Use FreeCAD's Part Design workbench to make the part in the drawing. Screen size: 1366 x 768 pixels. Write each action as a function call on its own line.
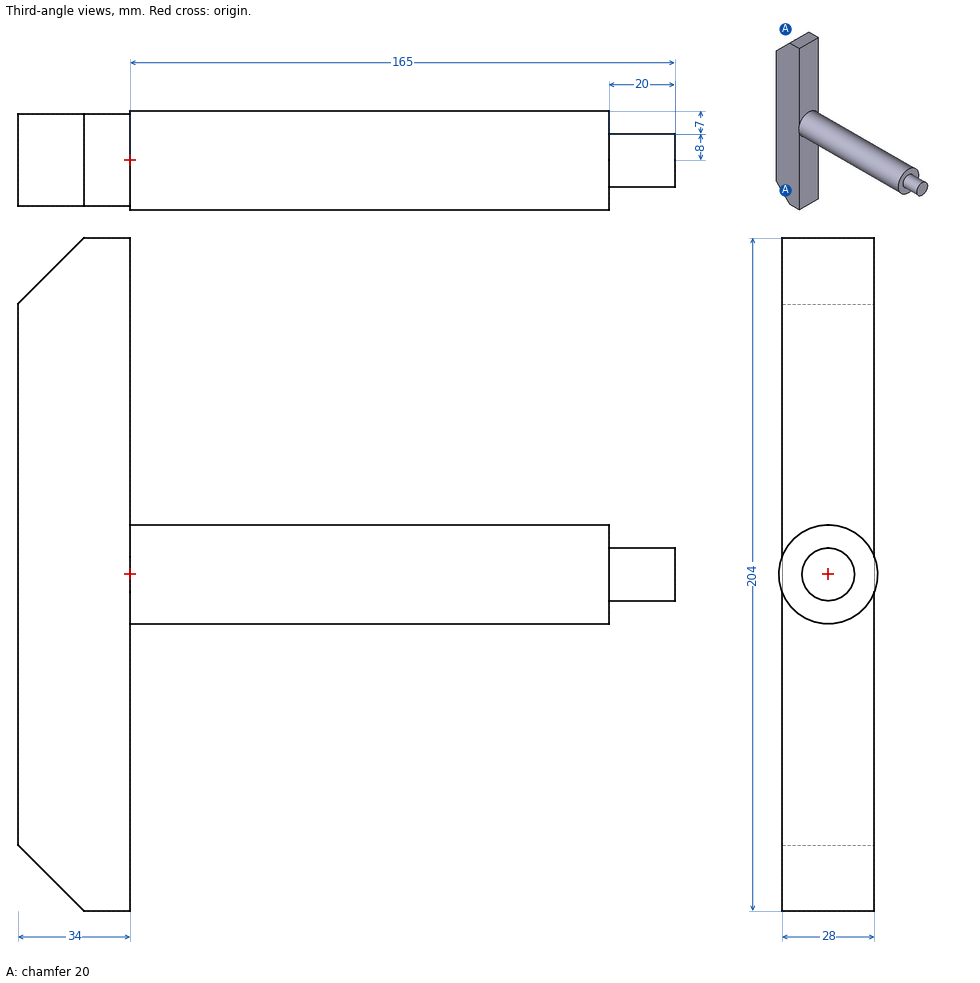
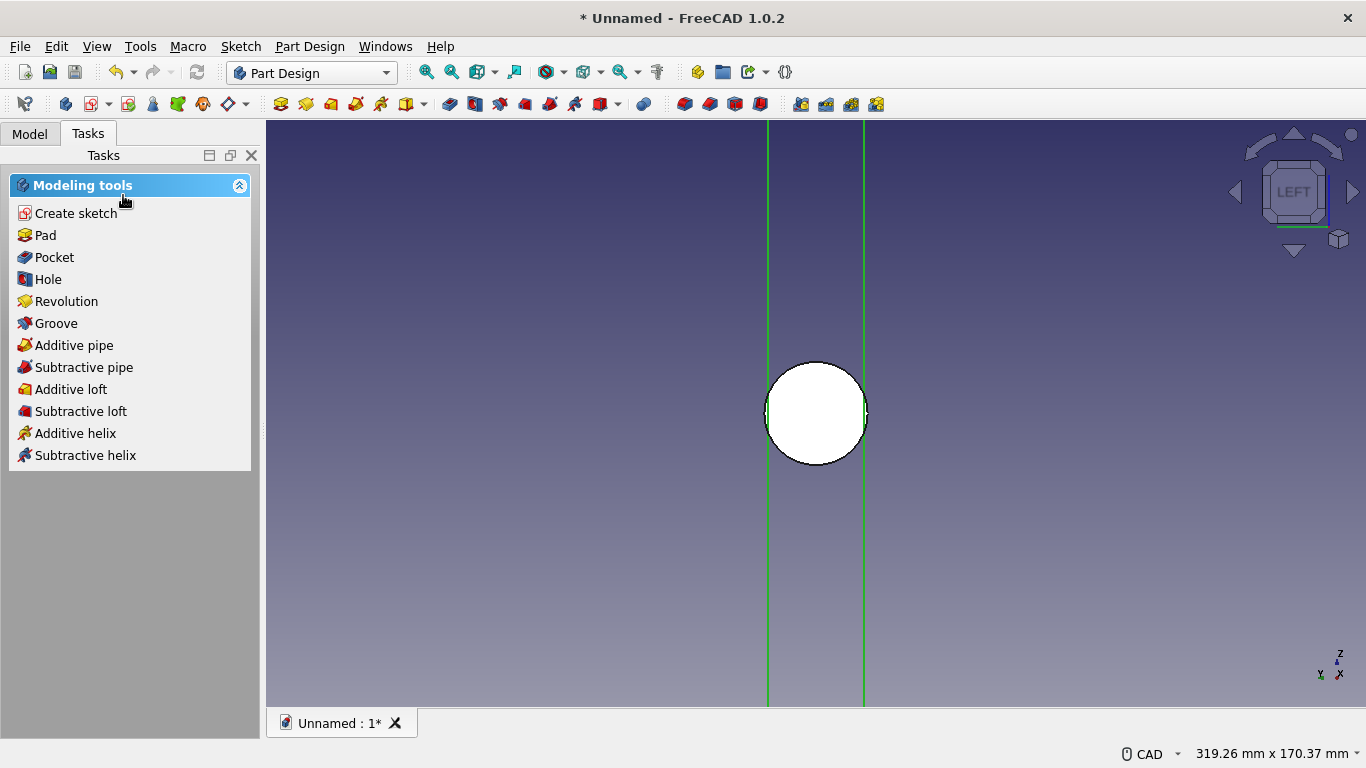
click(281, 104)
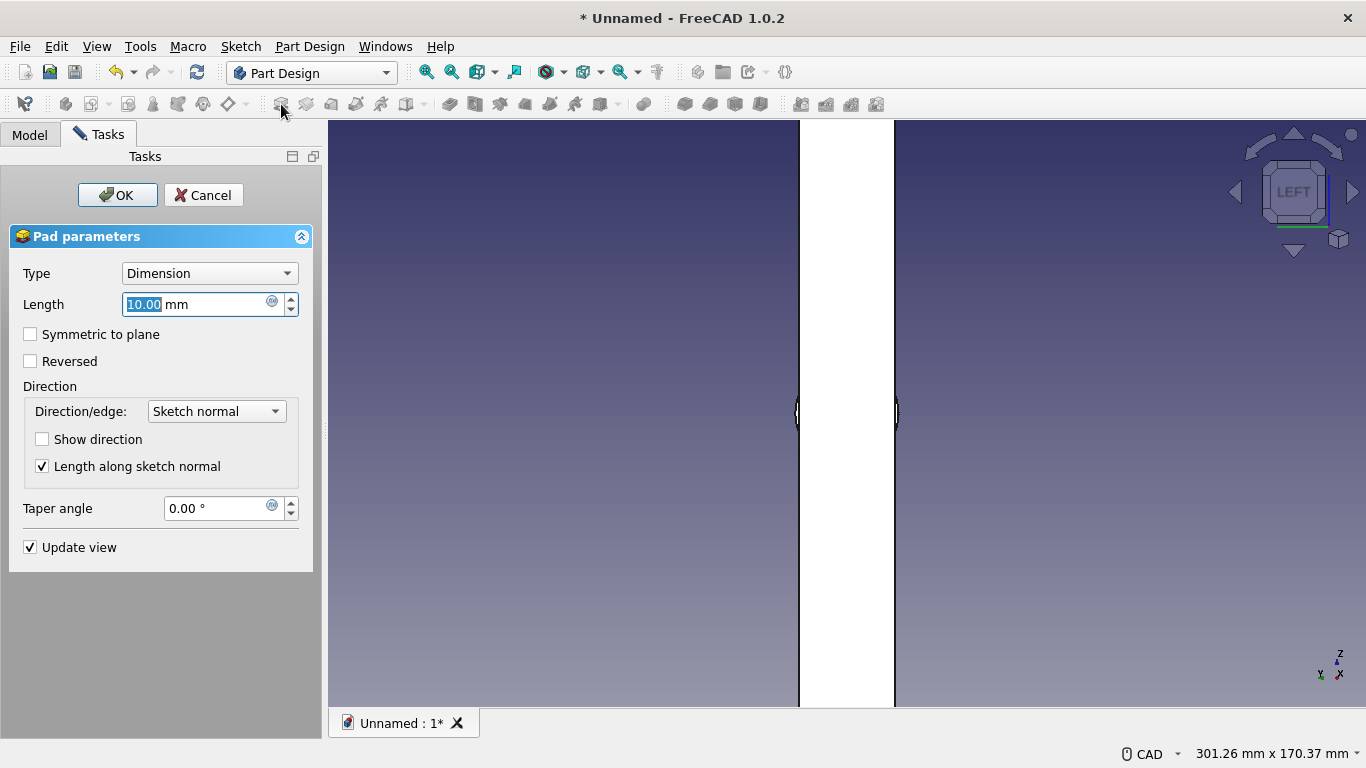
text(34)
key(Tab)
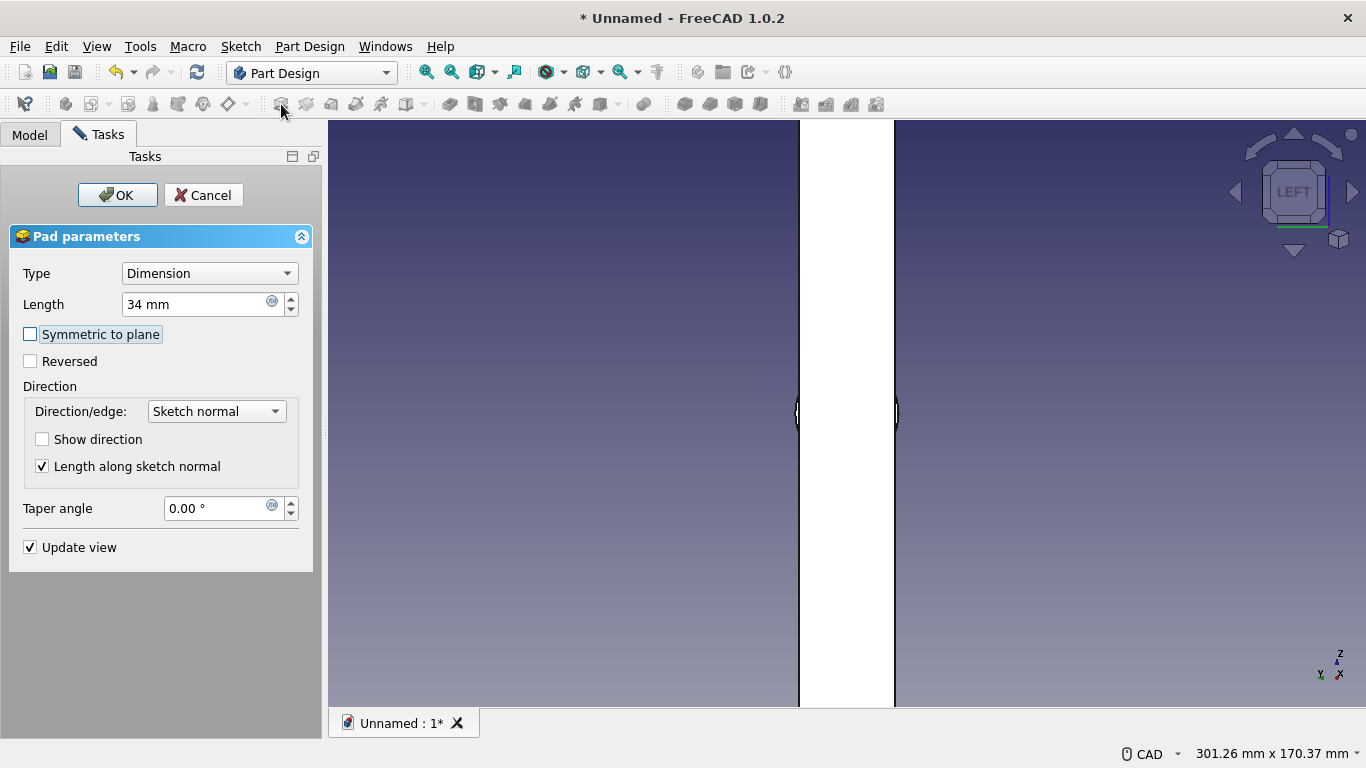
click(118, 195)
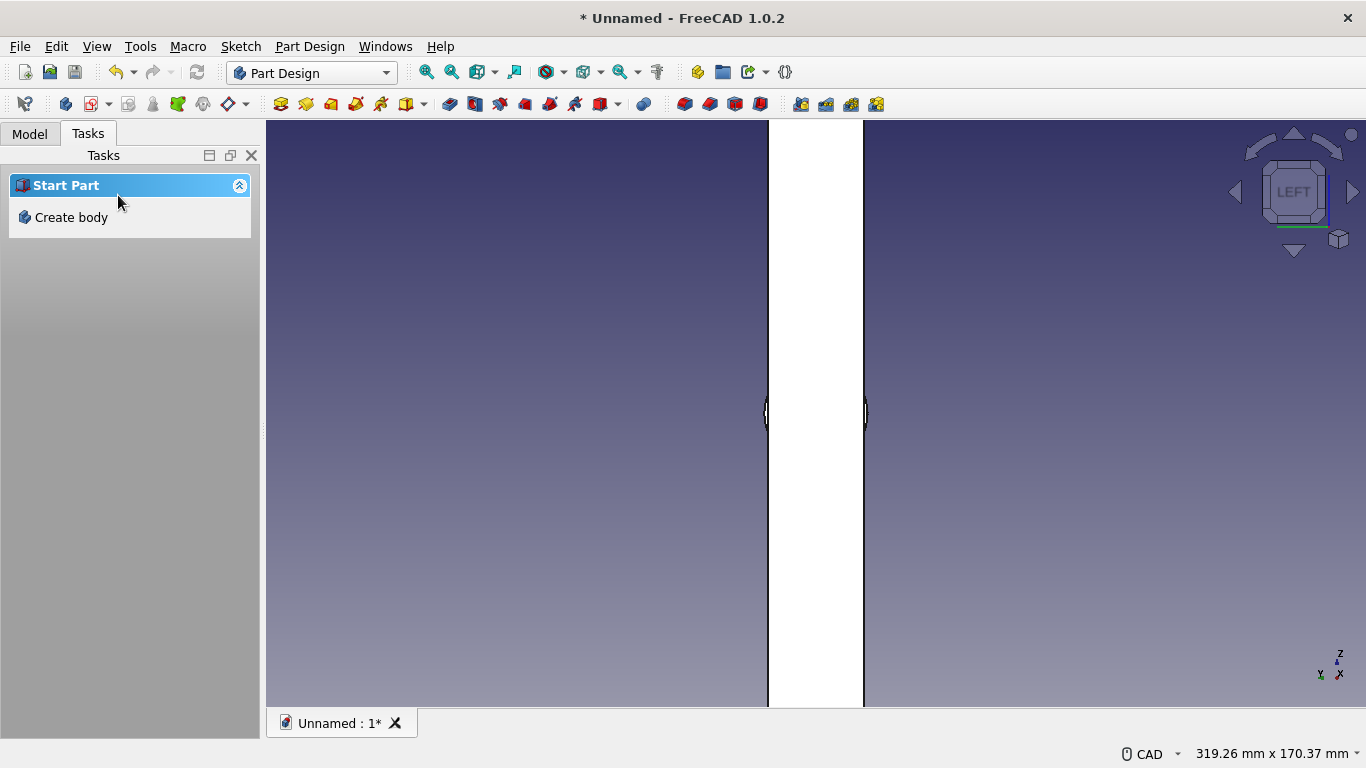
click(427, 72)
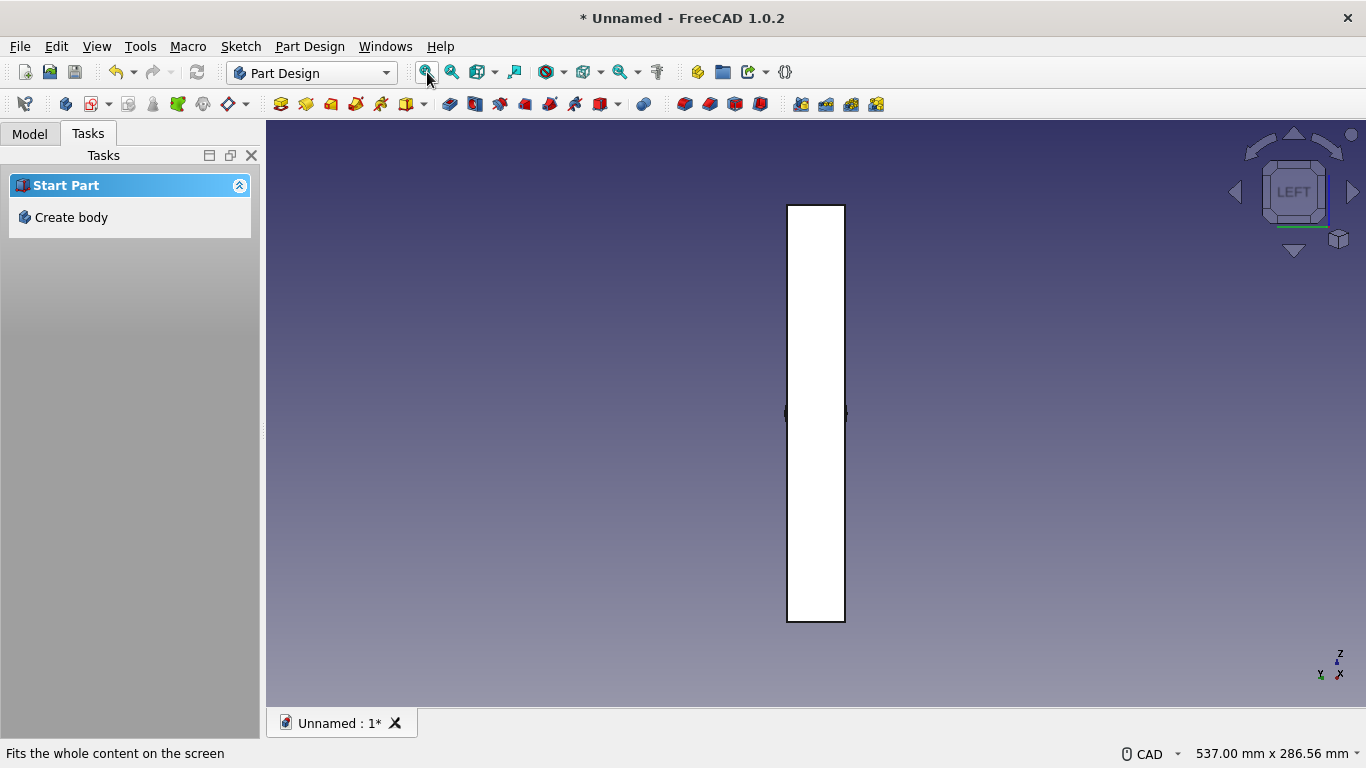
click(816, 621)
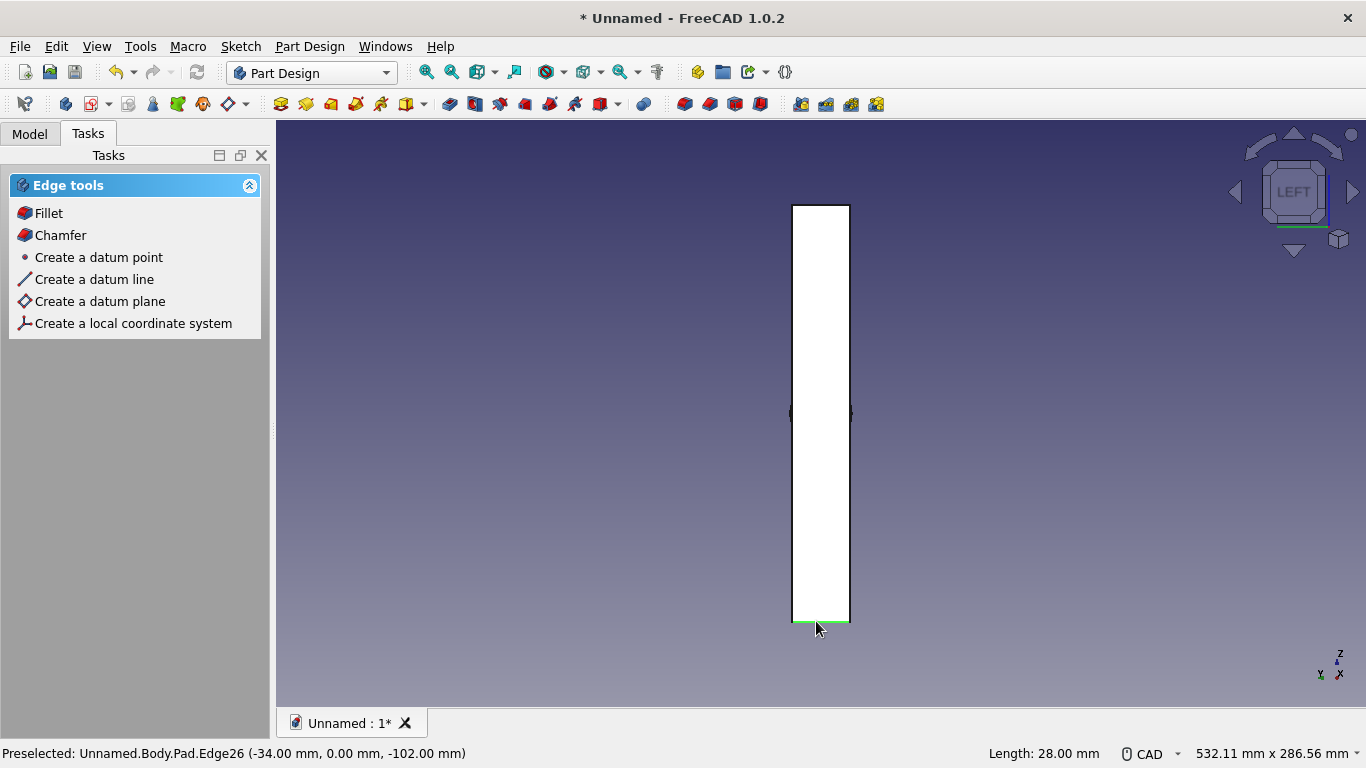
click(821, 204, ctrl)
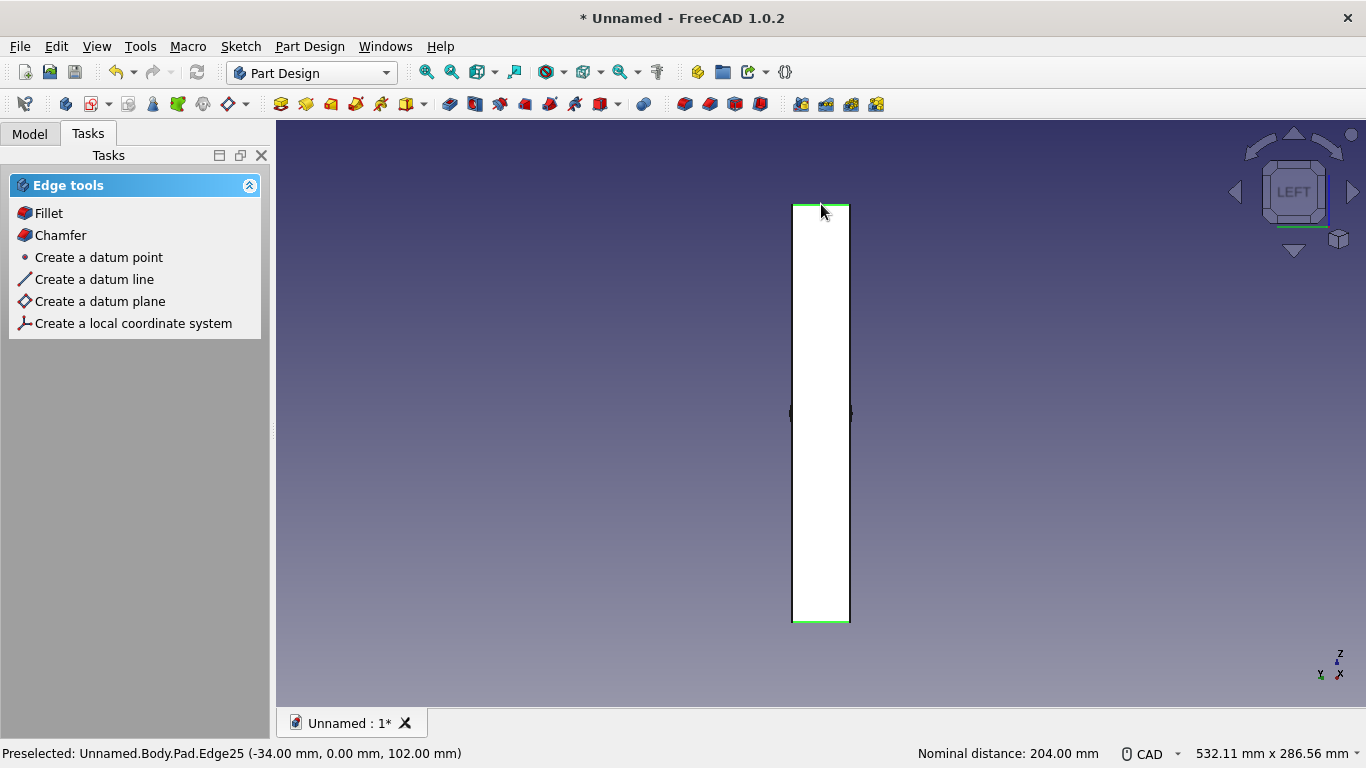
click(710, 104)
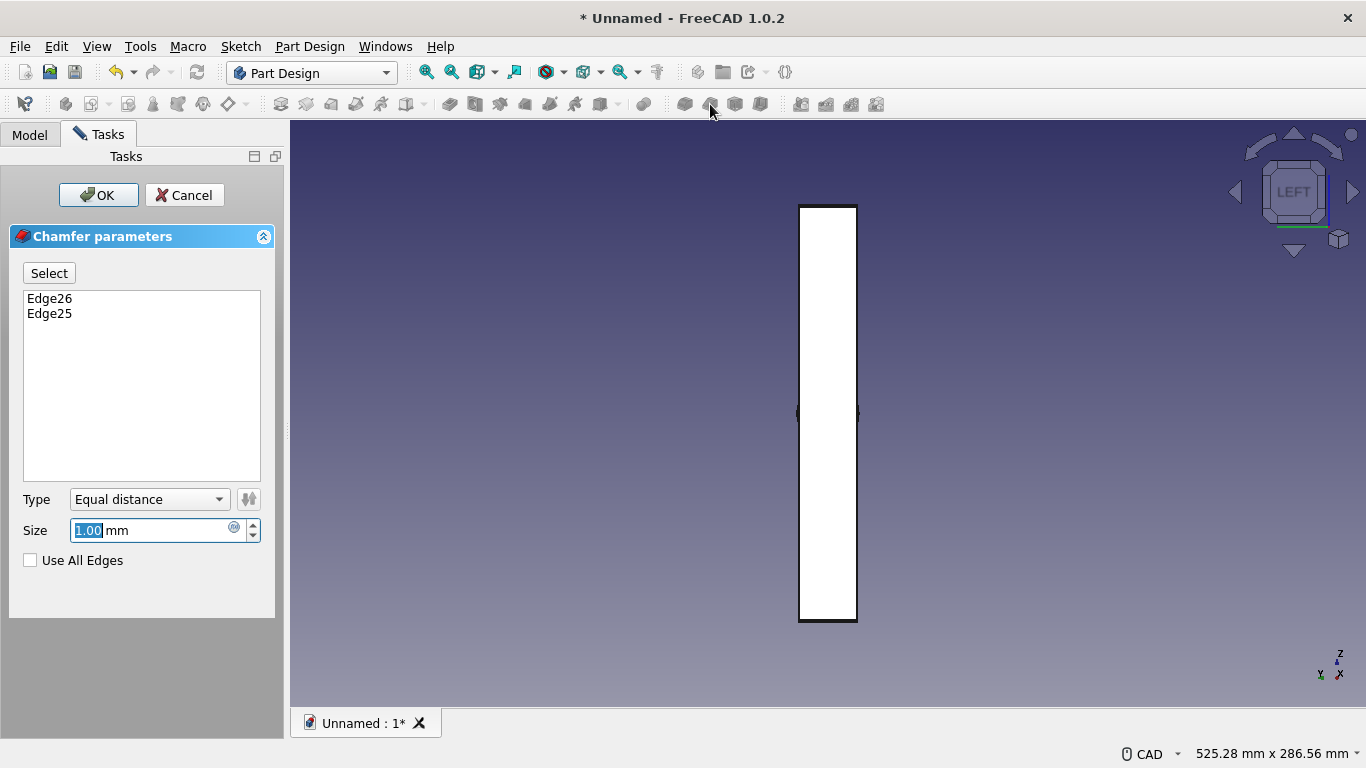
text(20)
key(Tab)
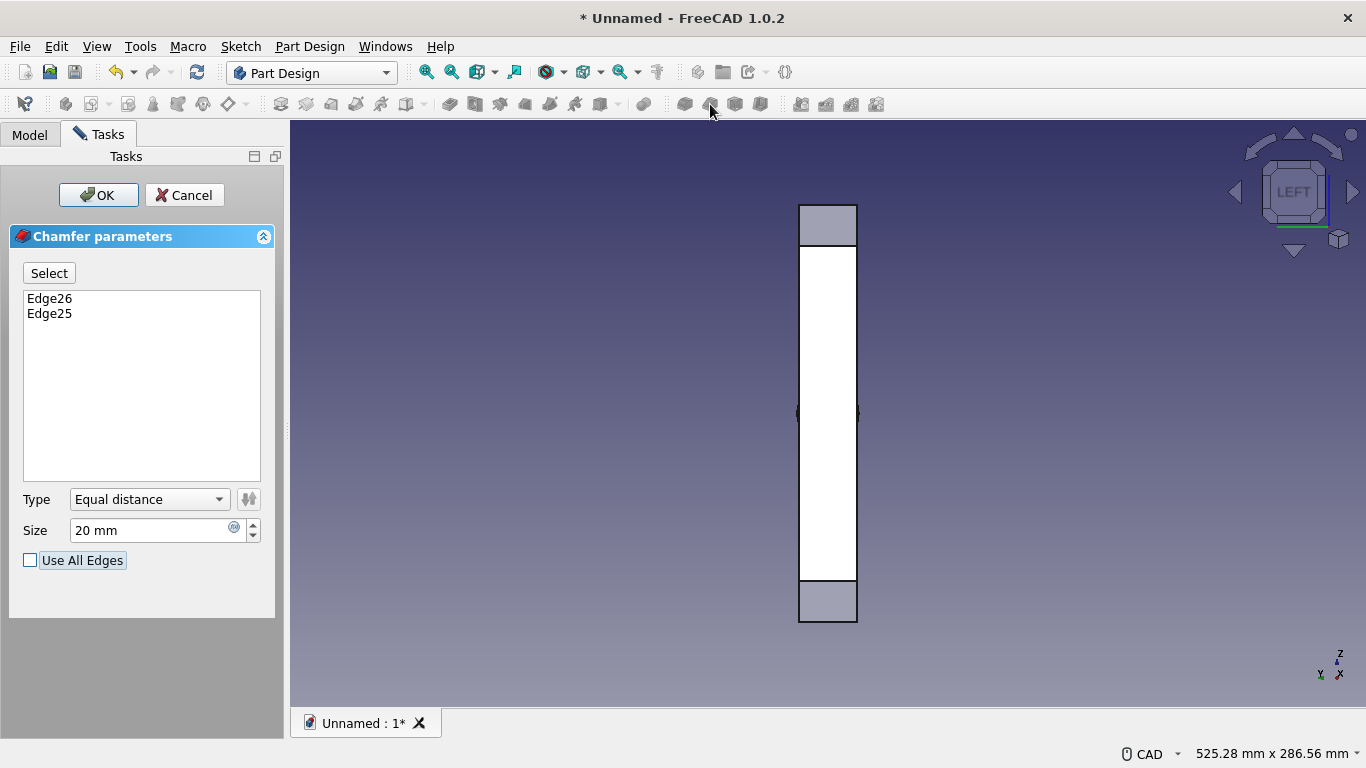
click(99, 195)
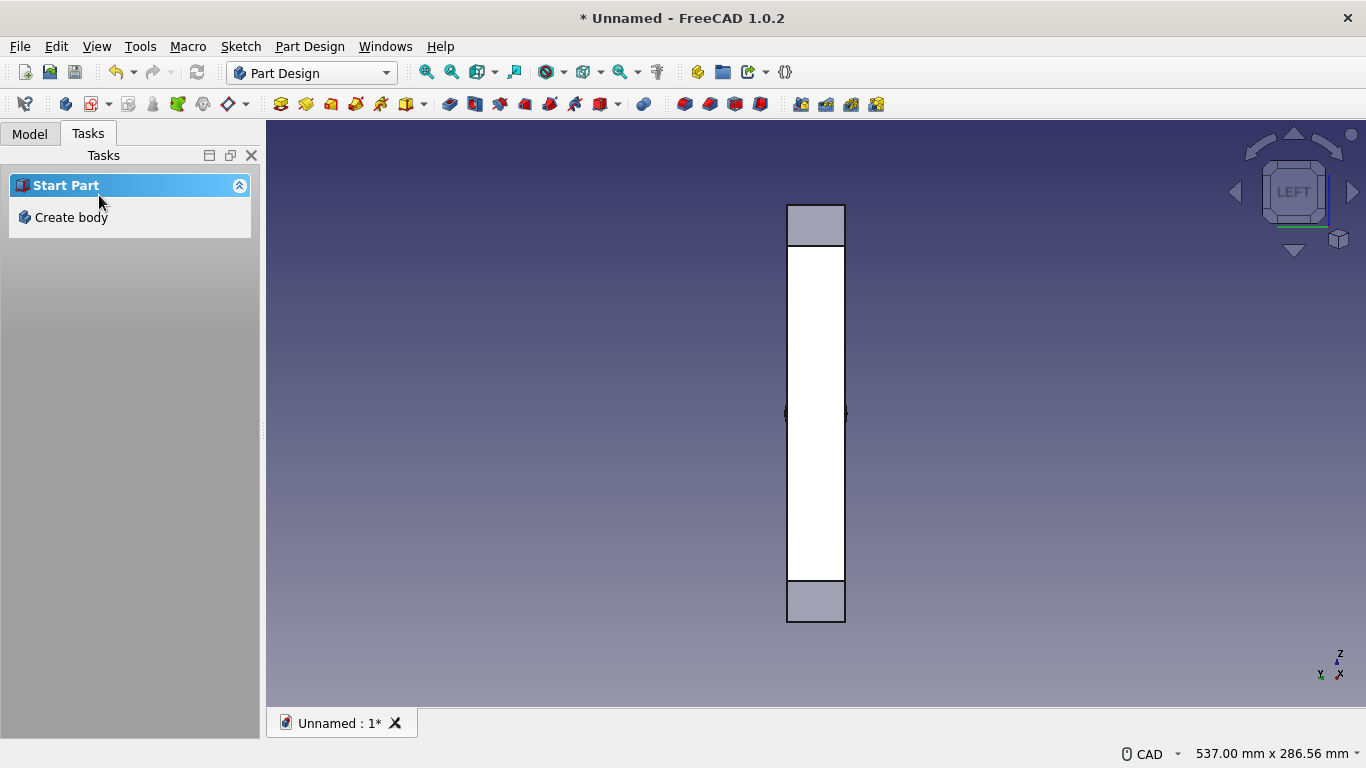
key(0)